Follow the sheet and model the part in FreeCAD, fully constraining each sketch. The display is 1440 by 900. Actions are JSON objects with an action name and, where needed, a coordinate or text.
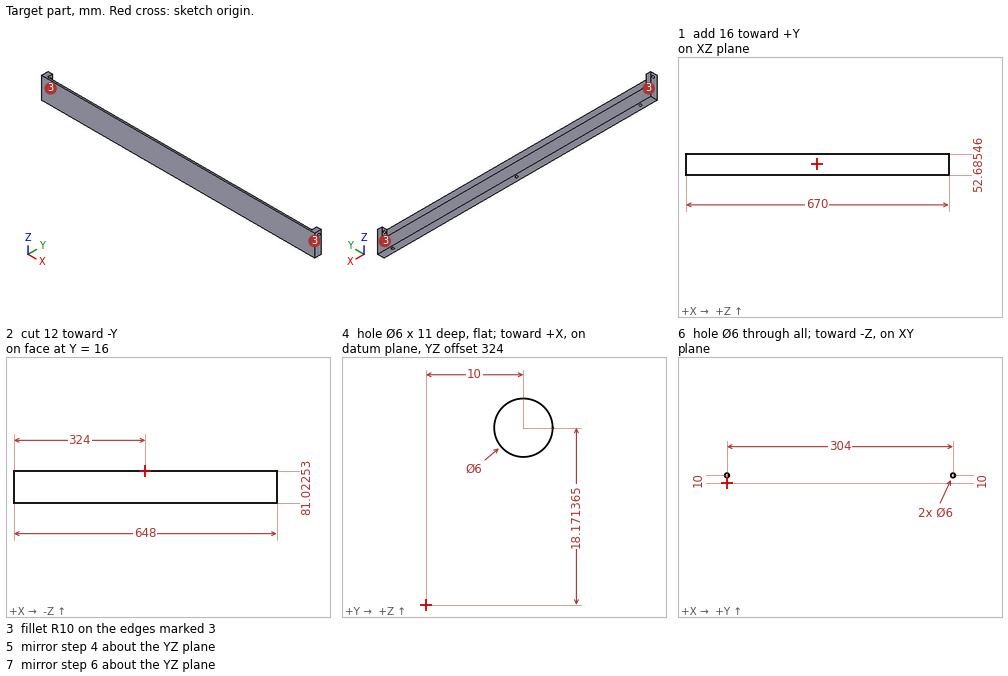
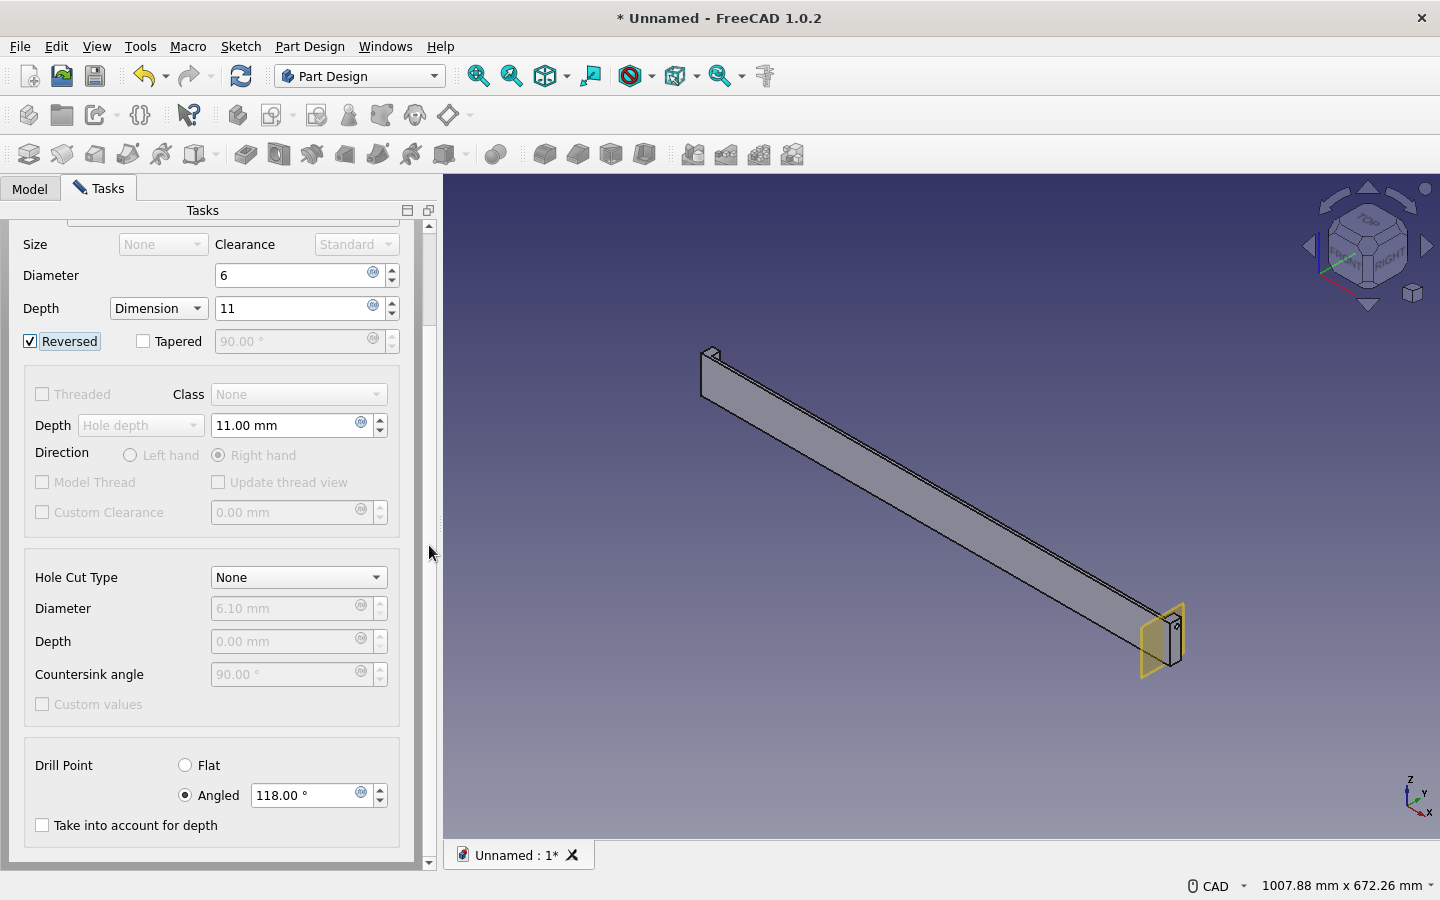
{"action": "left_click", "coordinate": [186, 763]}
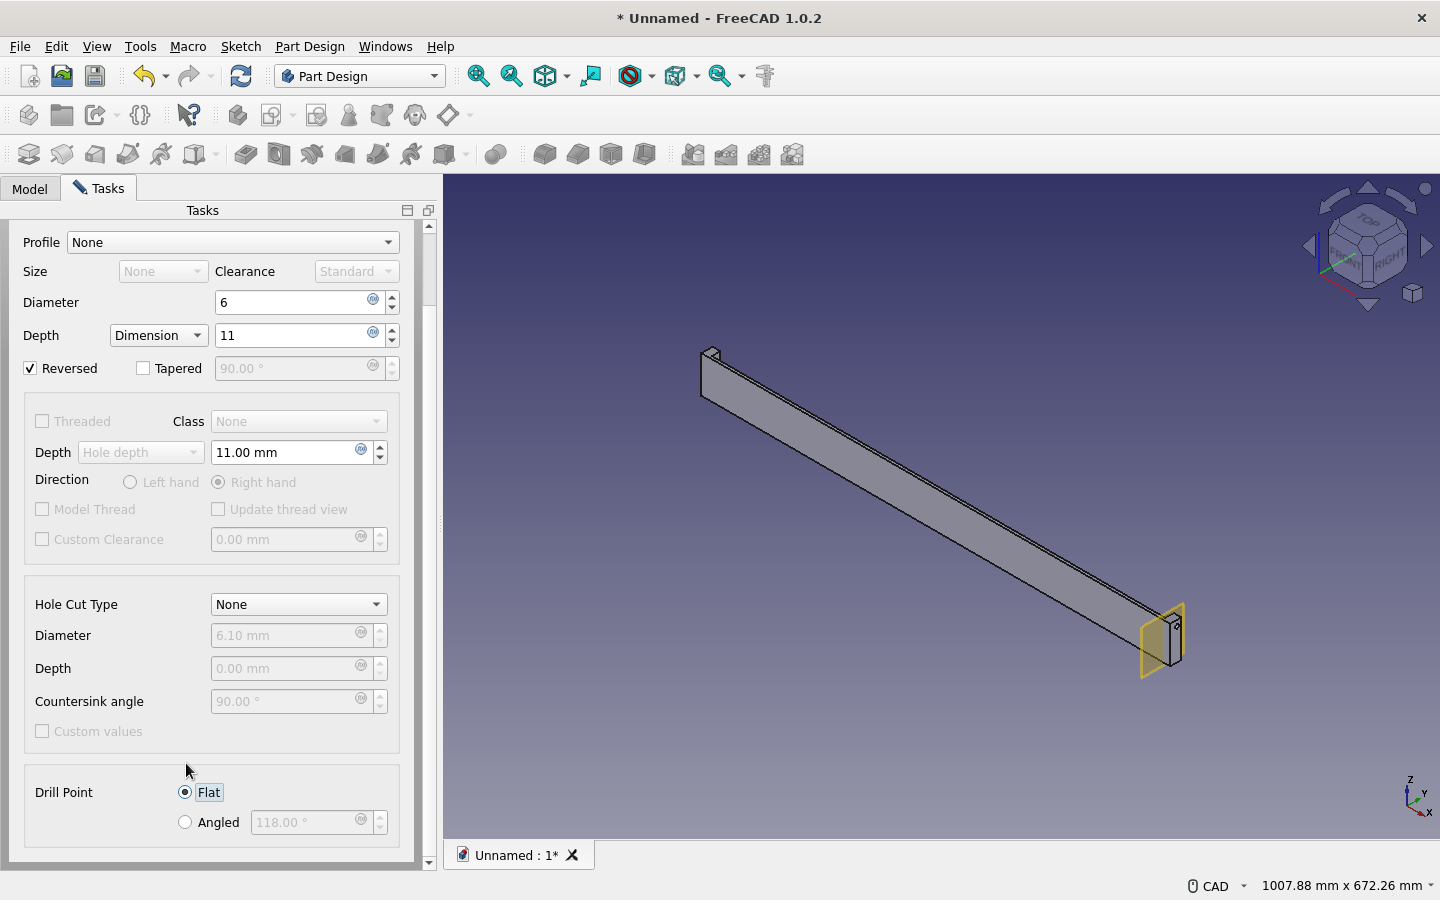
{"action": "scroll", "coordinate": [429, 545], "scroll_direction": "up", "scroll_amount": 3}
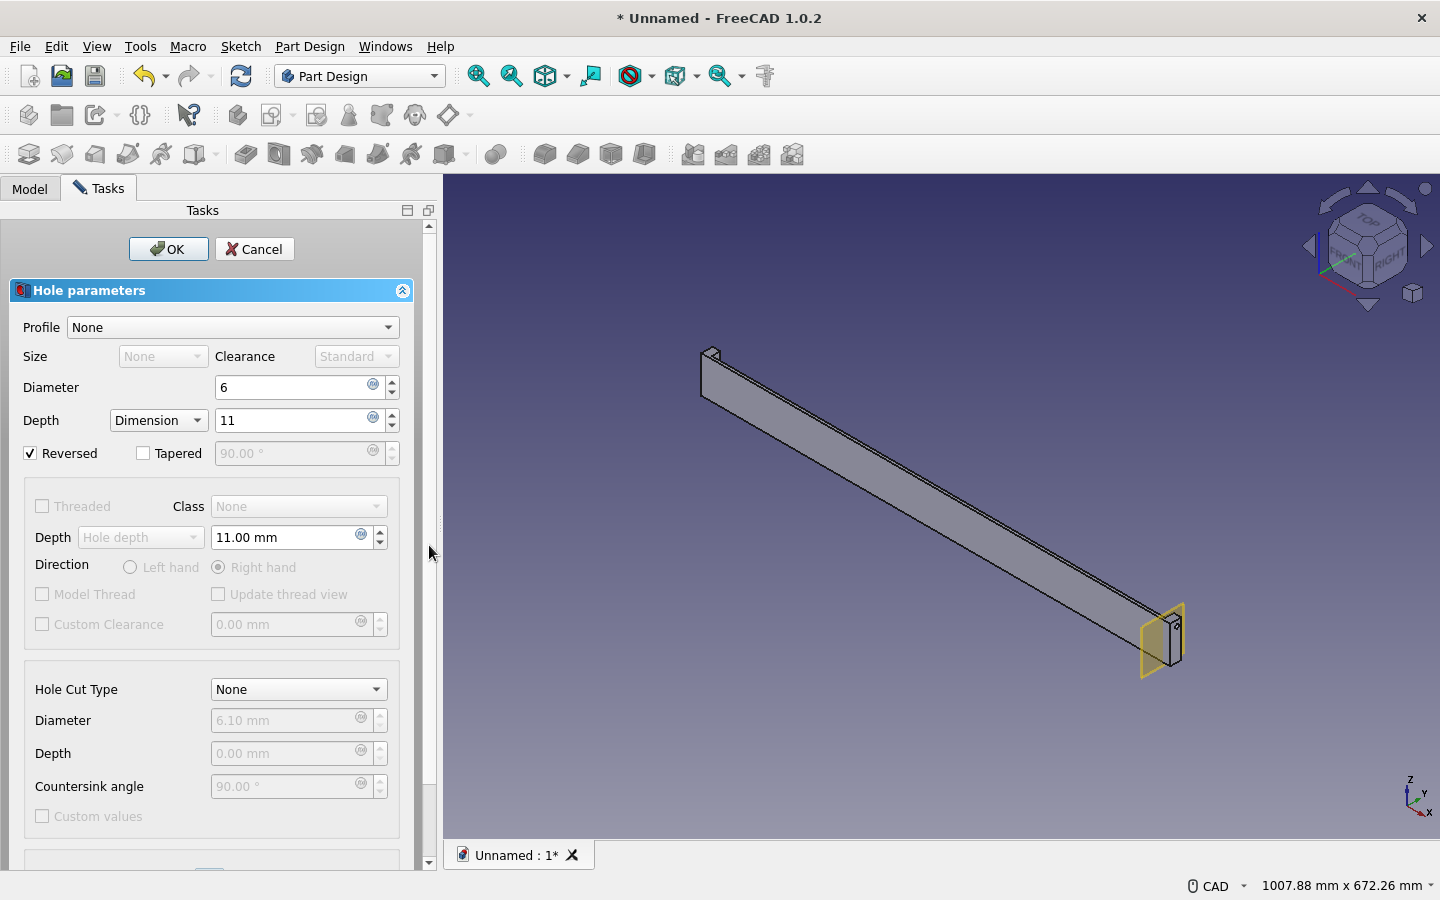
{"action": "left_click", "coordinate": [169, 249]}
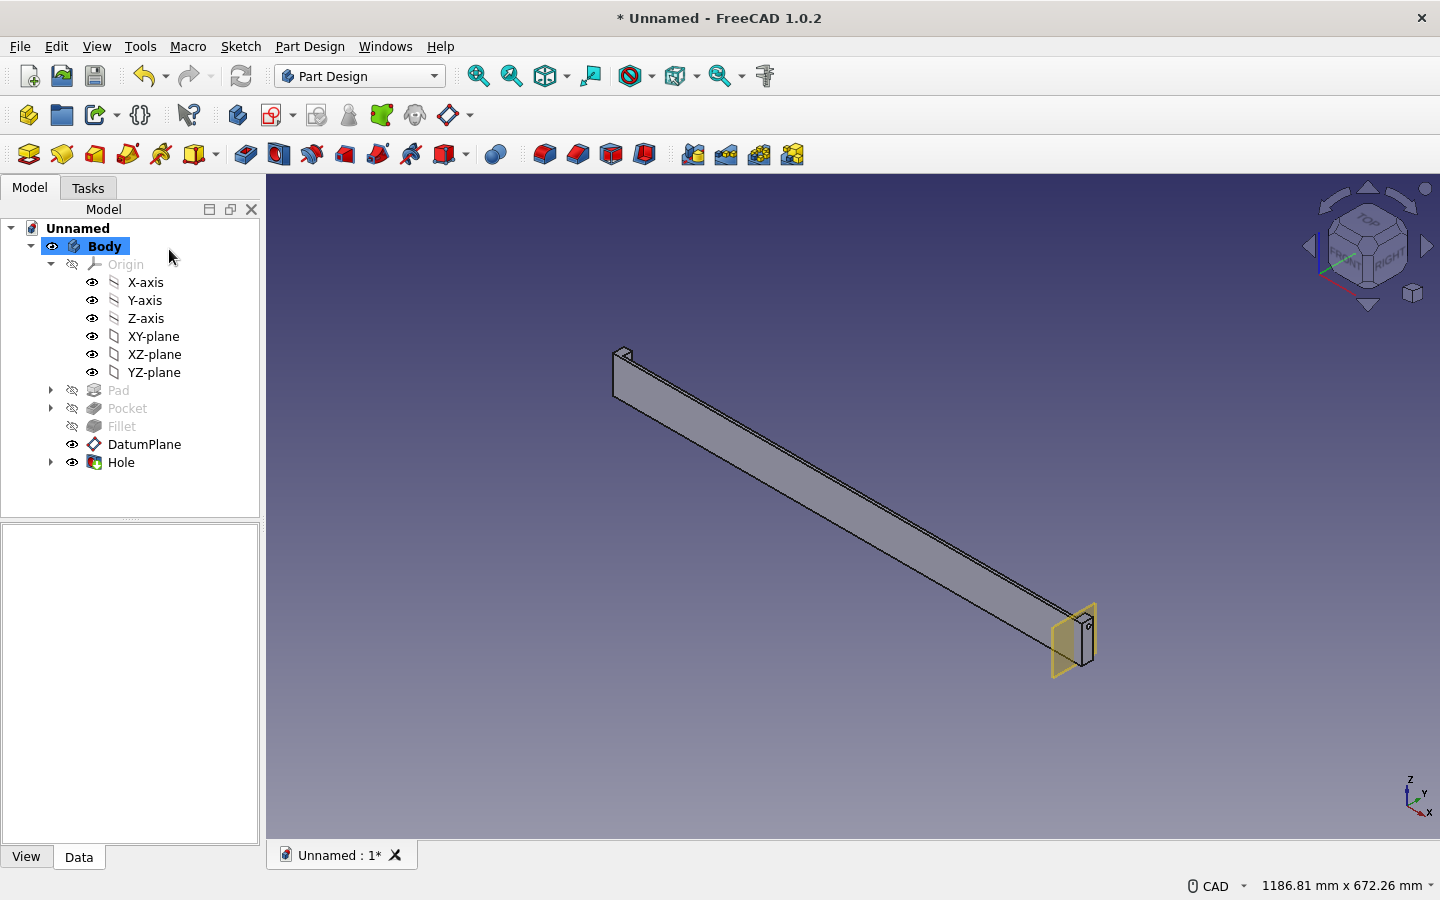
{"action": "left_click", "coordinate": [117, 444]}
{"action": "key", "text": "space"}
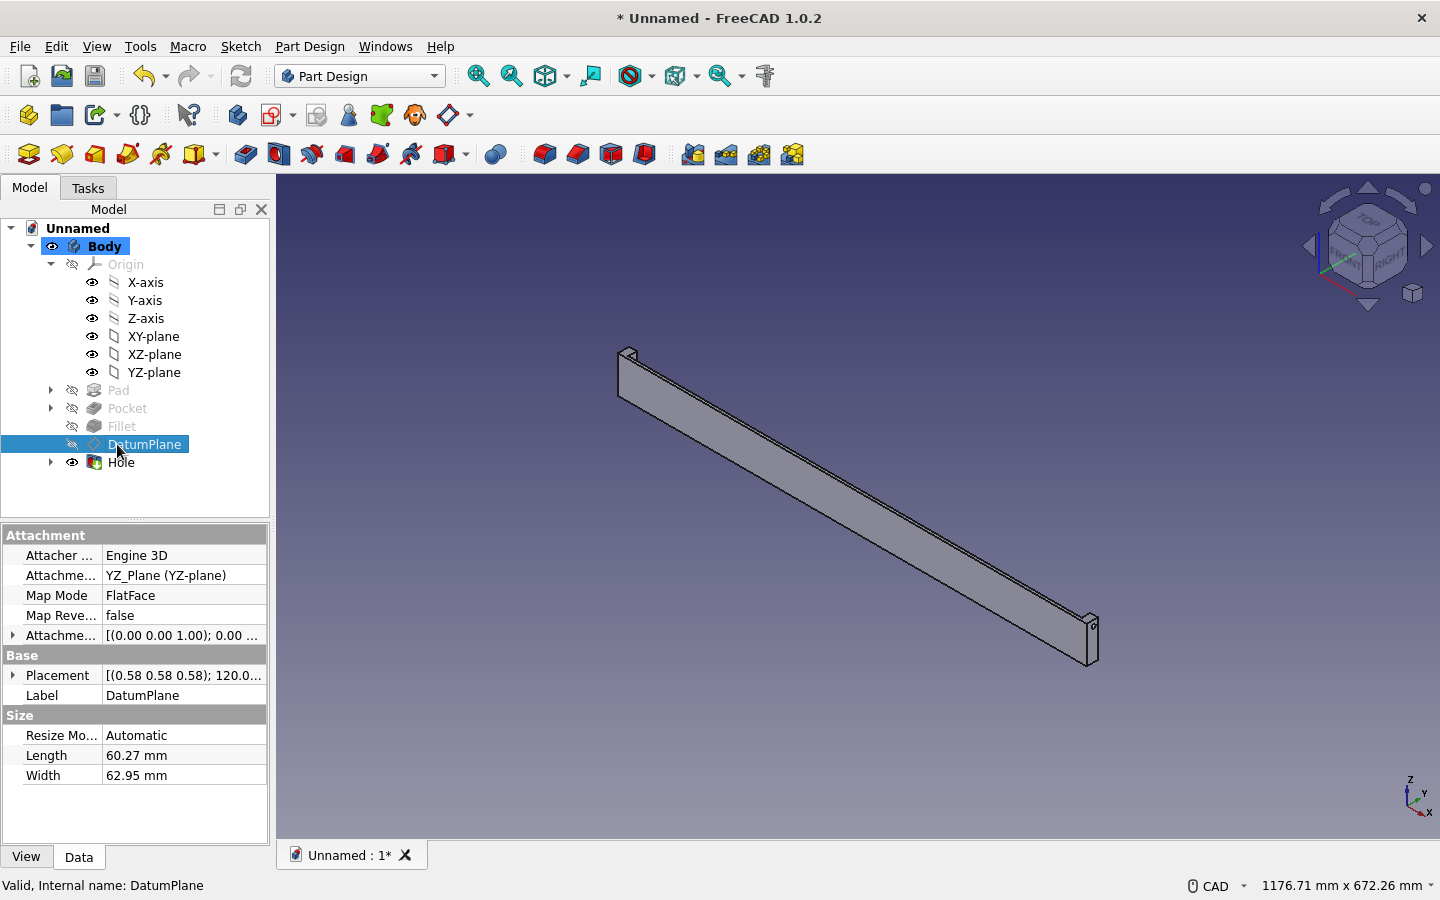
{"action": "left_click", "coordinate": [117, 462]}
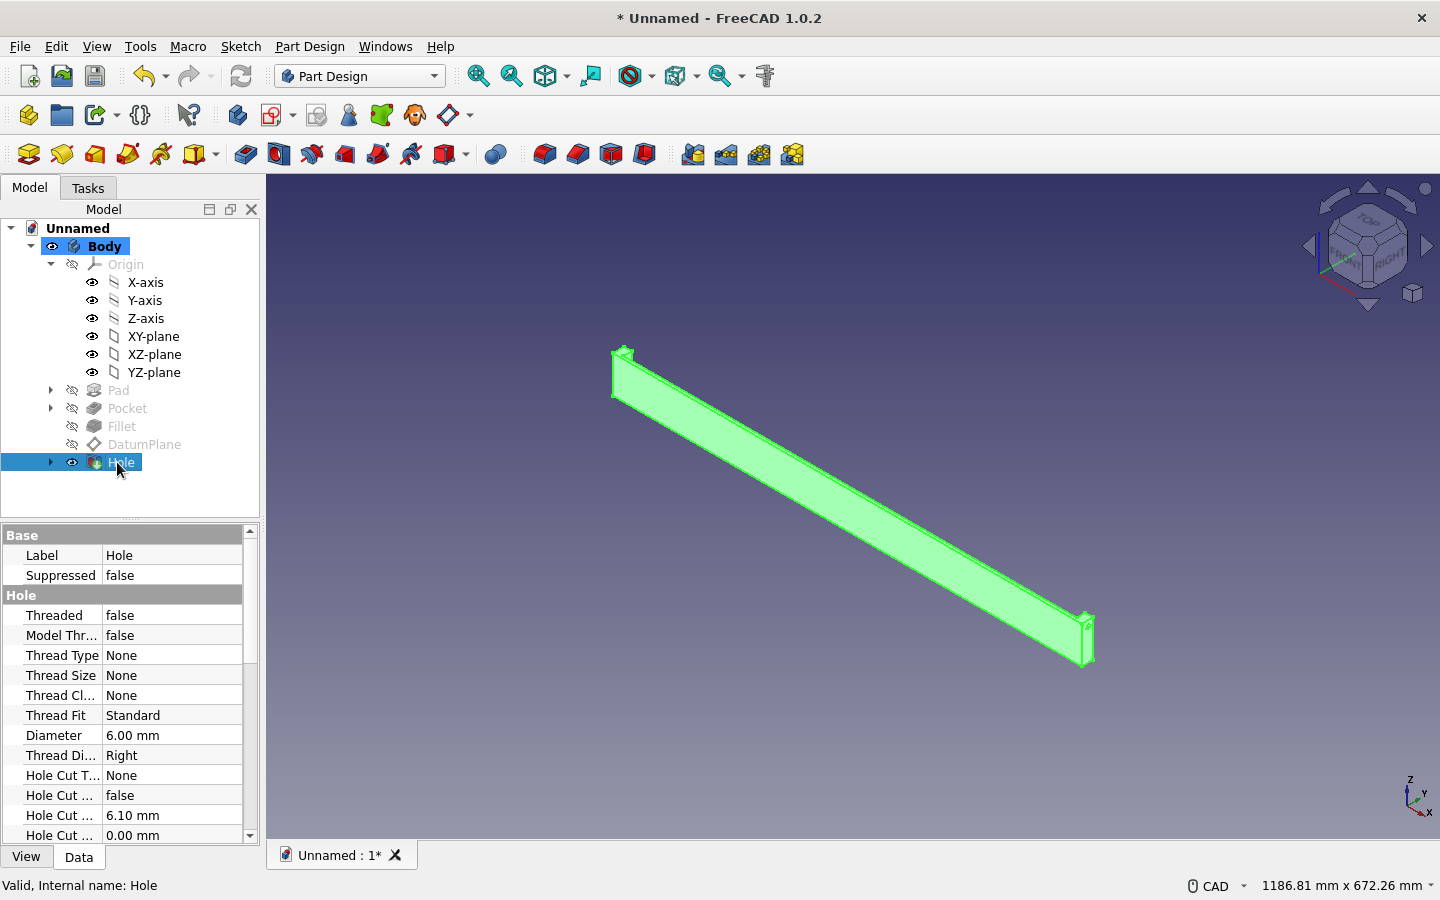
{"action": "left_click", "coordinate": [693, 154]}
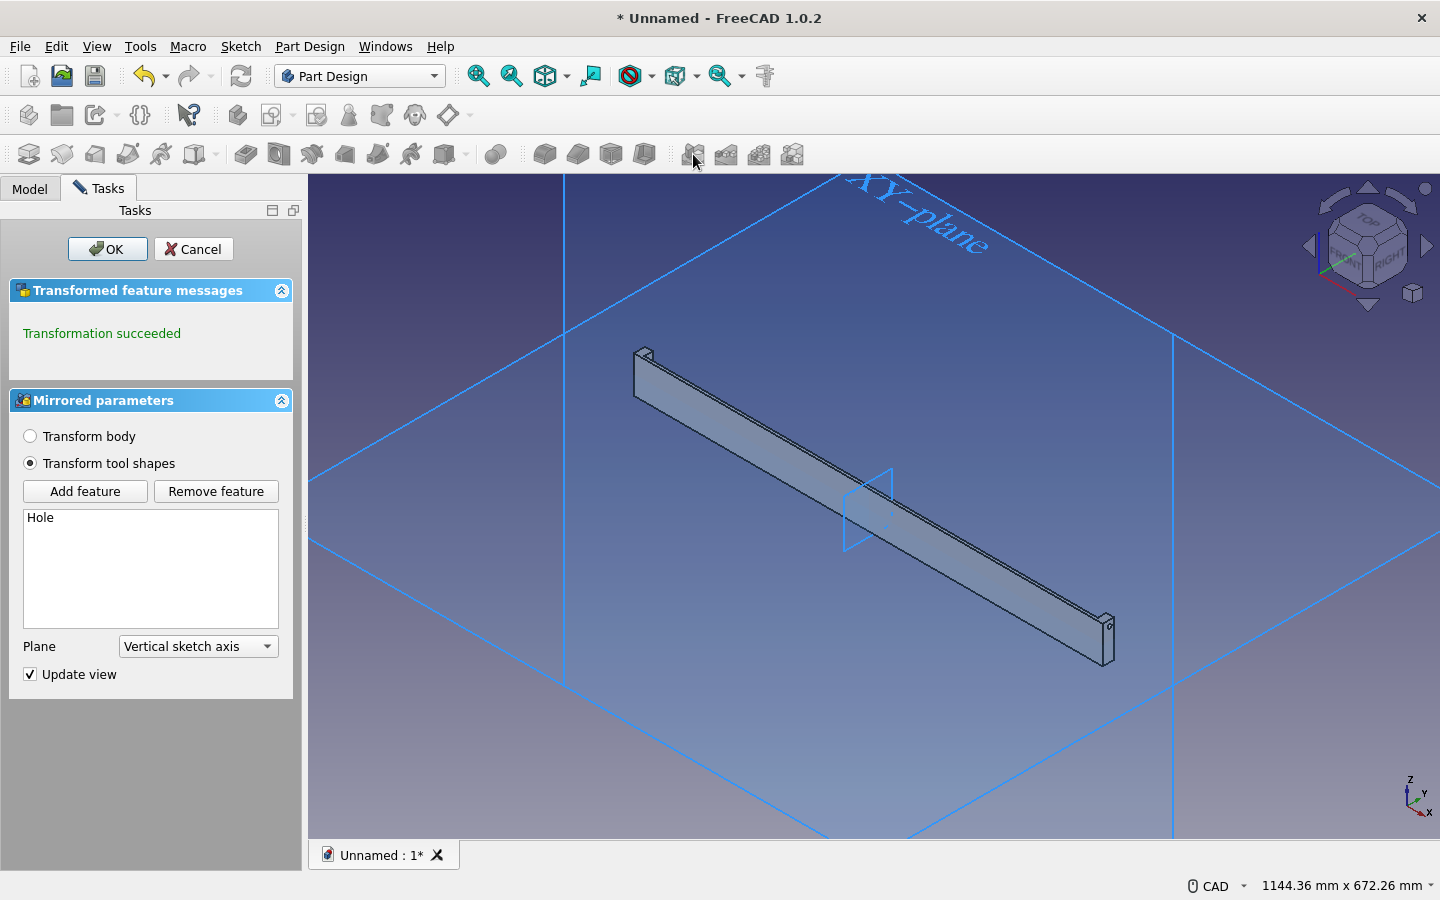
{"action": "left_click", "coordinate": [199, 646]}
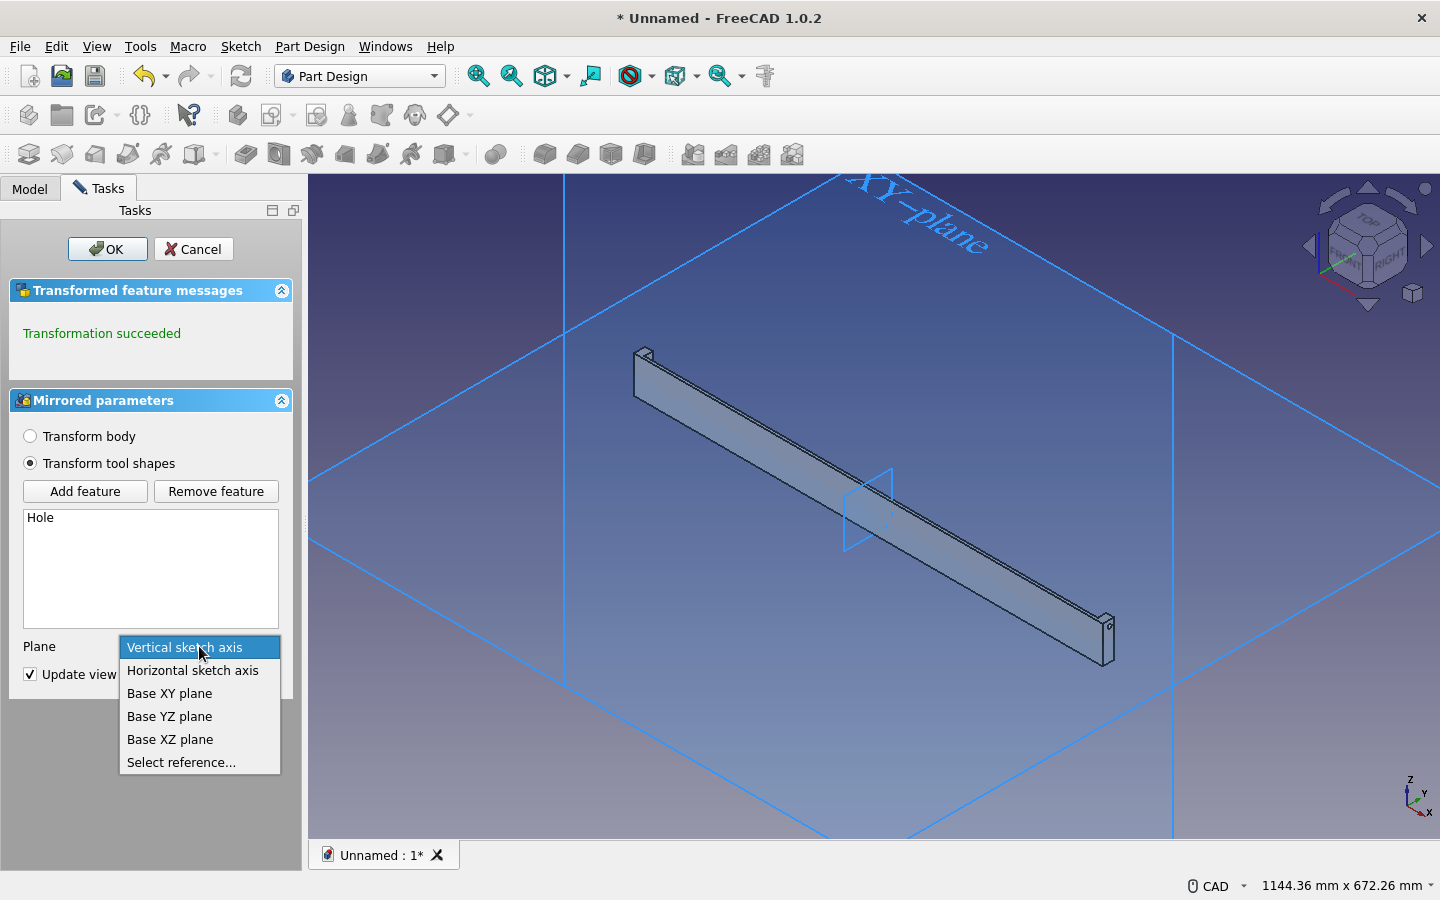
{"action": "left_click", "coordinate": [198, 716]}